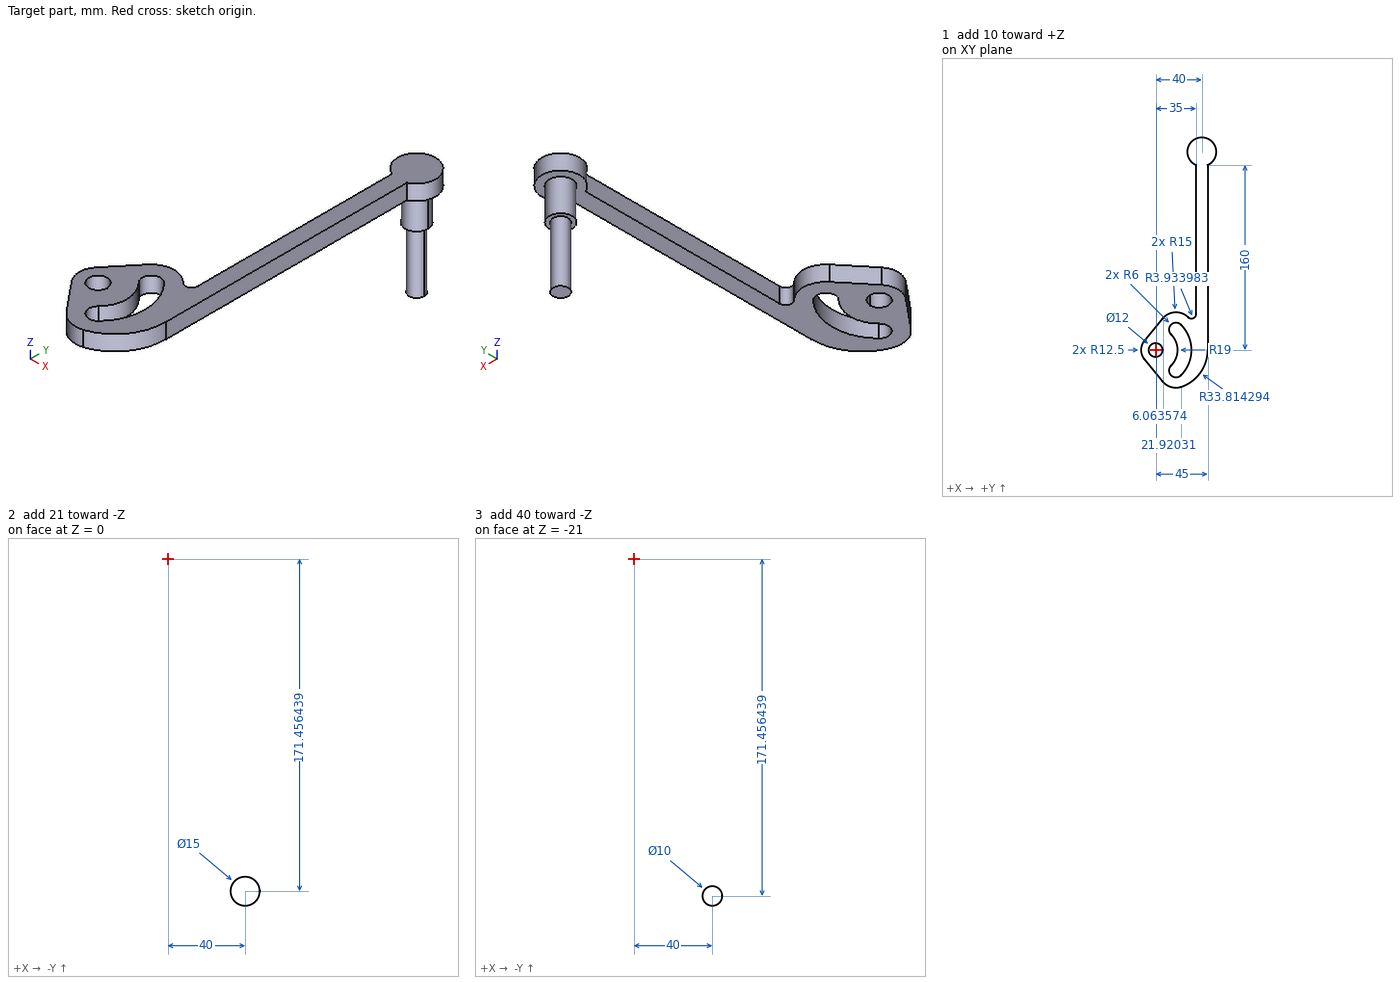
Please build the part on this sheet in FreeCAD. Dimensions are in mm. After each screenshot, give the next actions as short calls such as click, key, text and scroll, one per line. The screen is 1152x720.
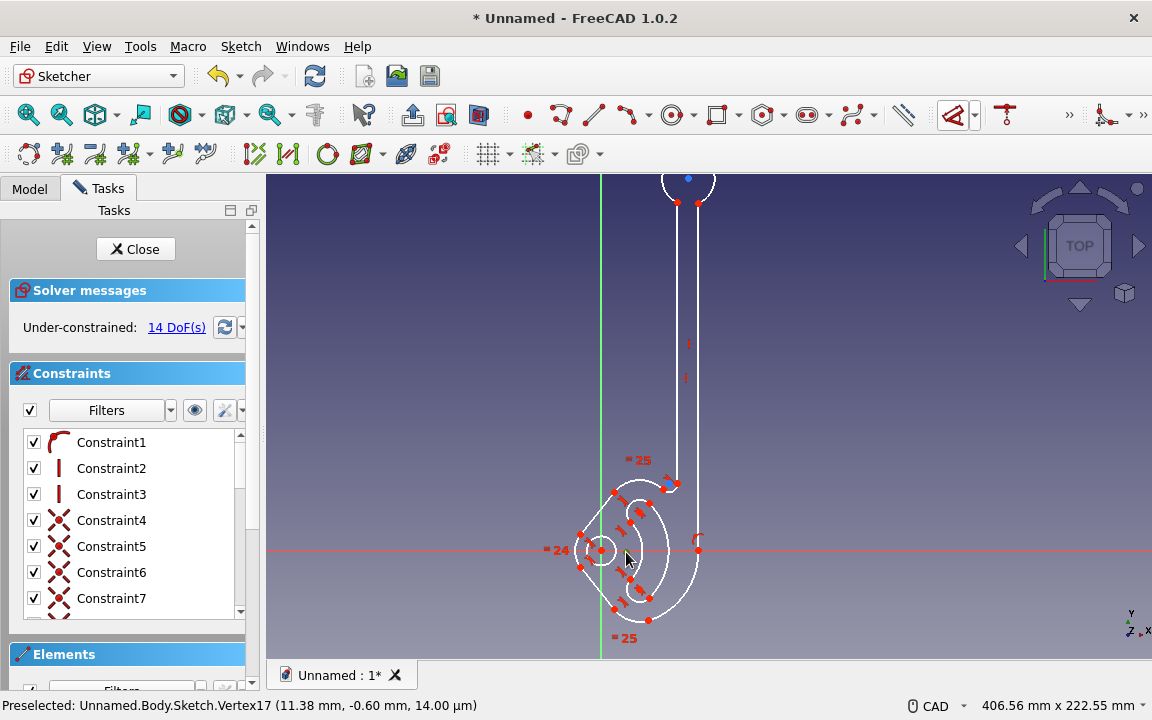
click(344, 551)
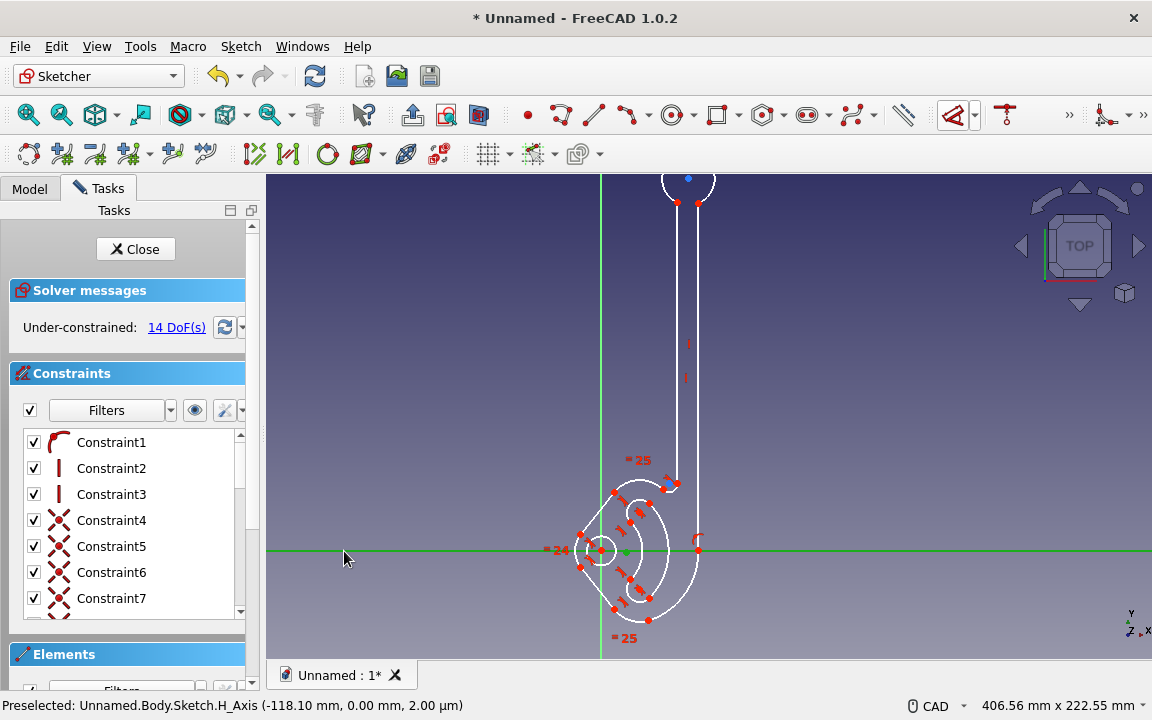
click(1005, 116)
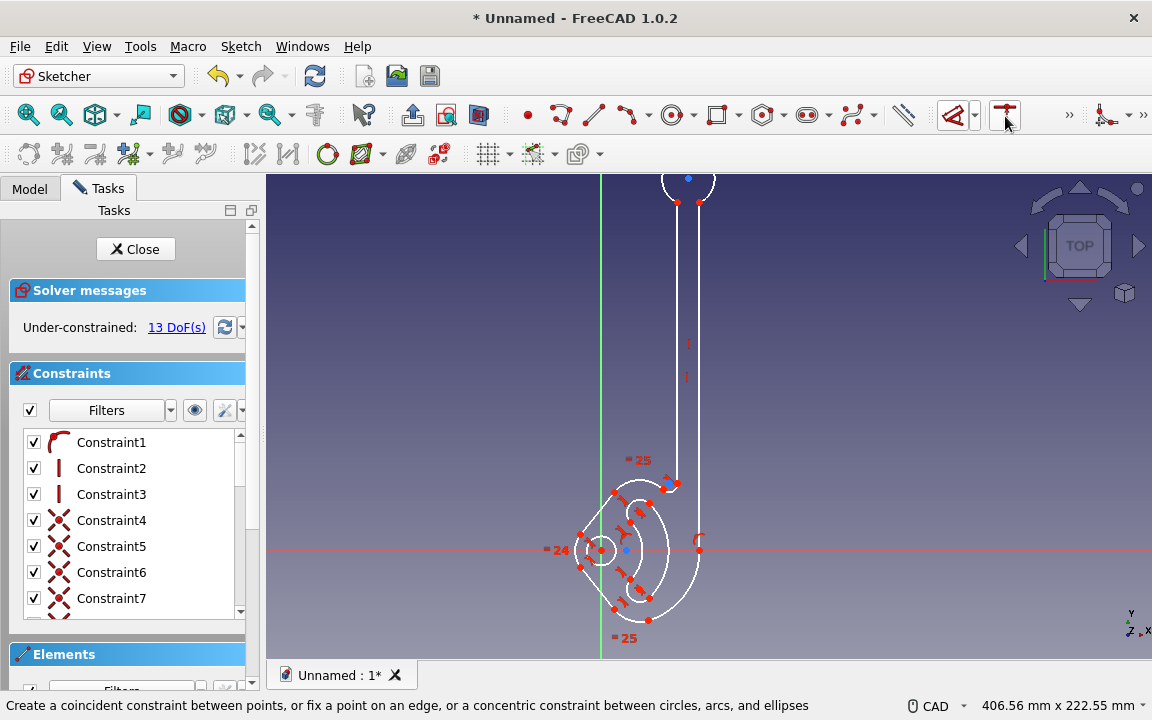
key(d)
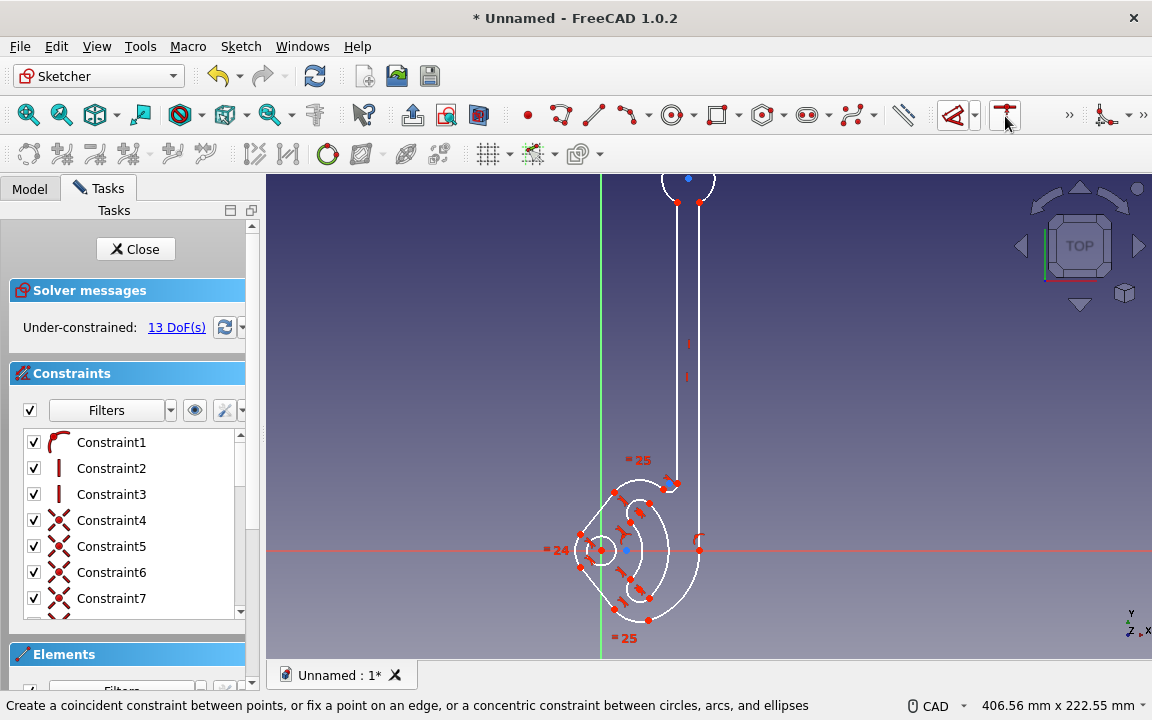
scroll(575, 551, up, 2)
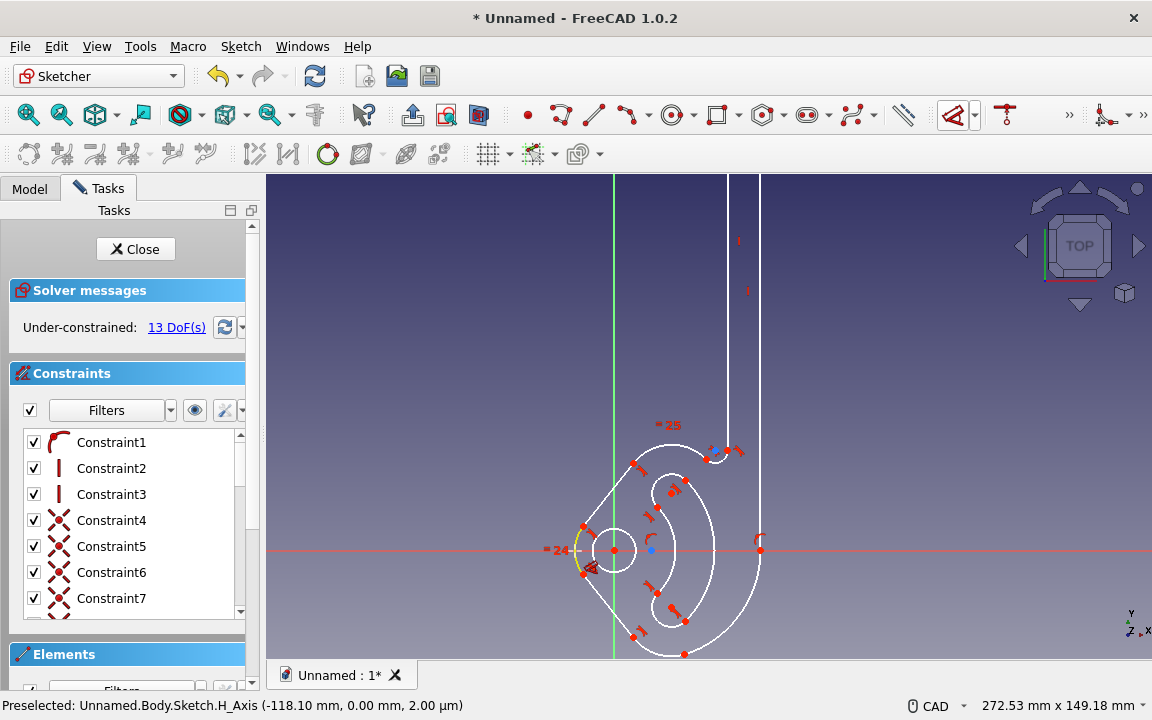
click(575, 551)
click(551, 517)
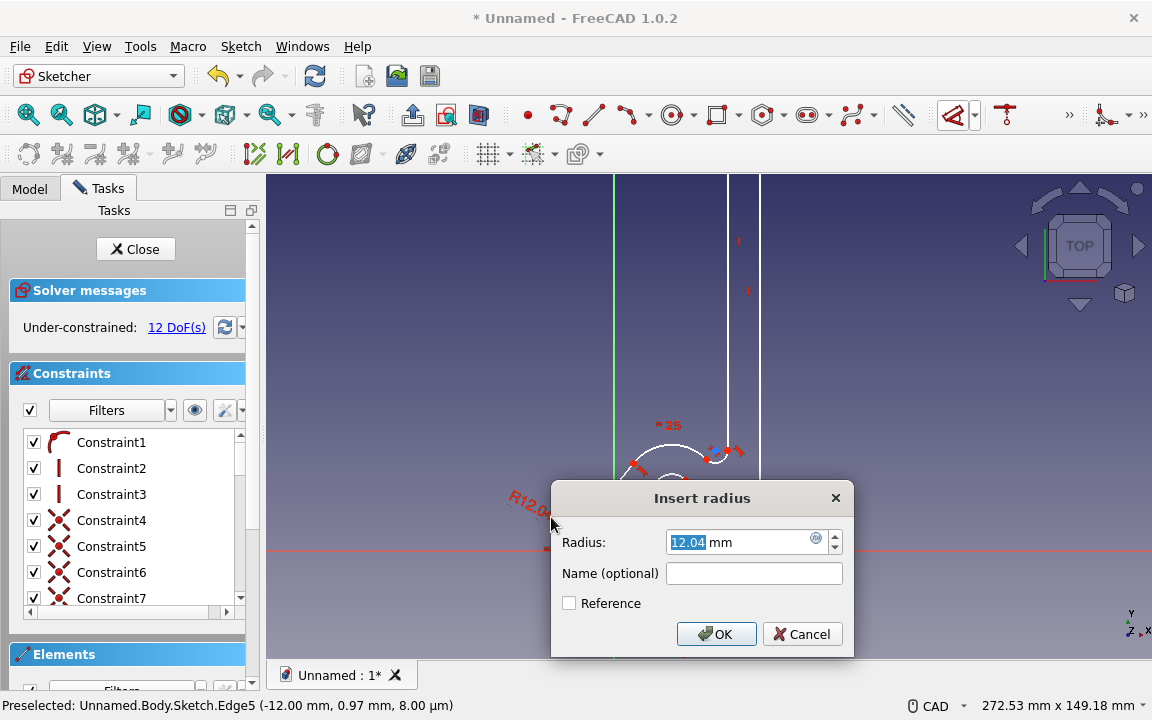
text(12.5)
key(Return)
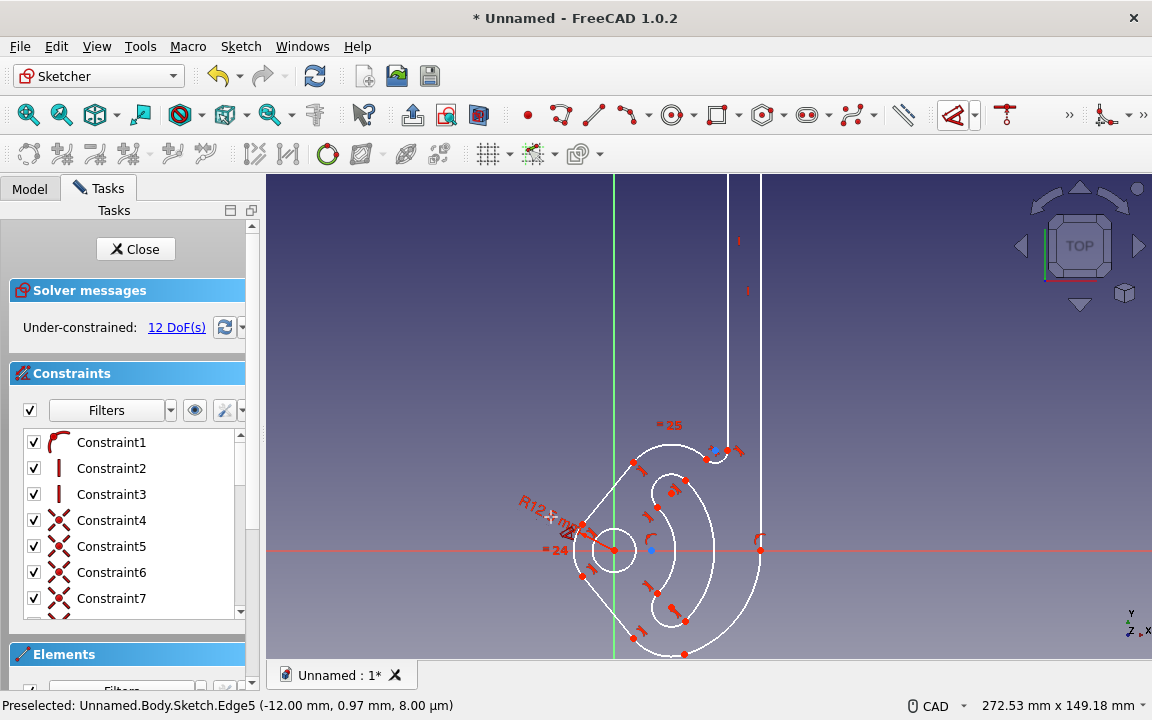
scroll(619, 509, down, 4)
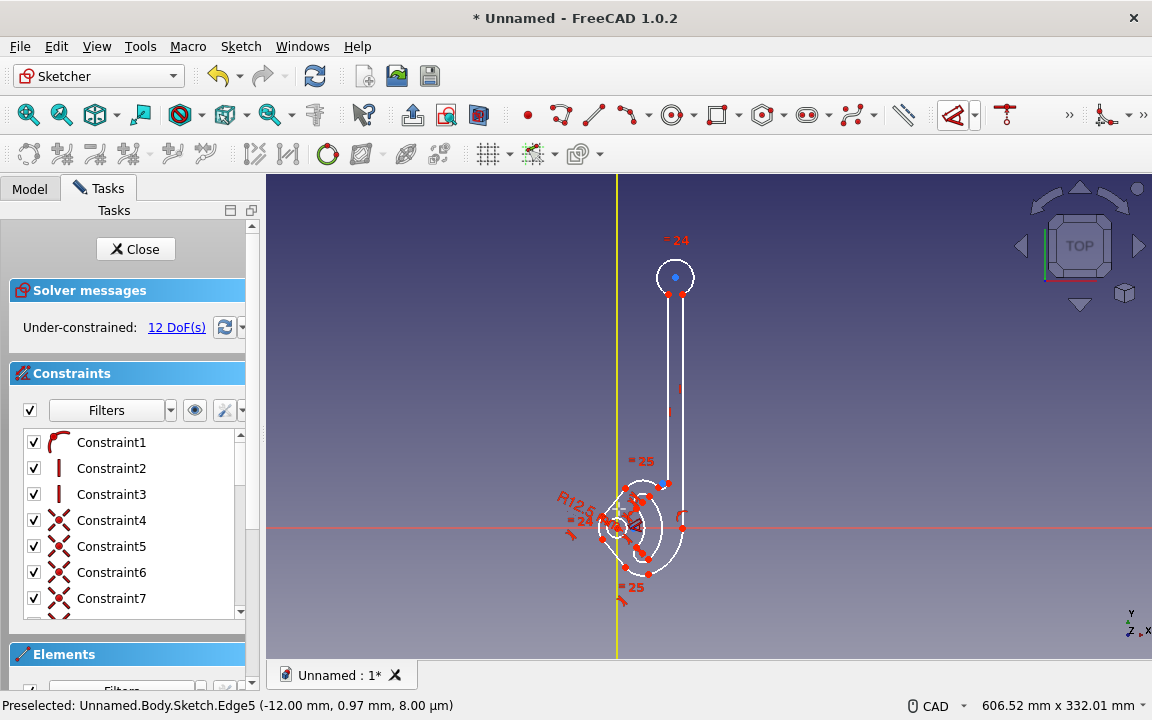
scroll(631, 573, up, 3)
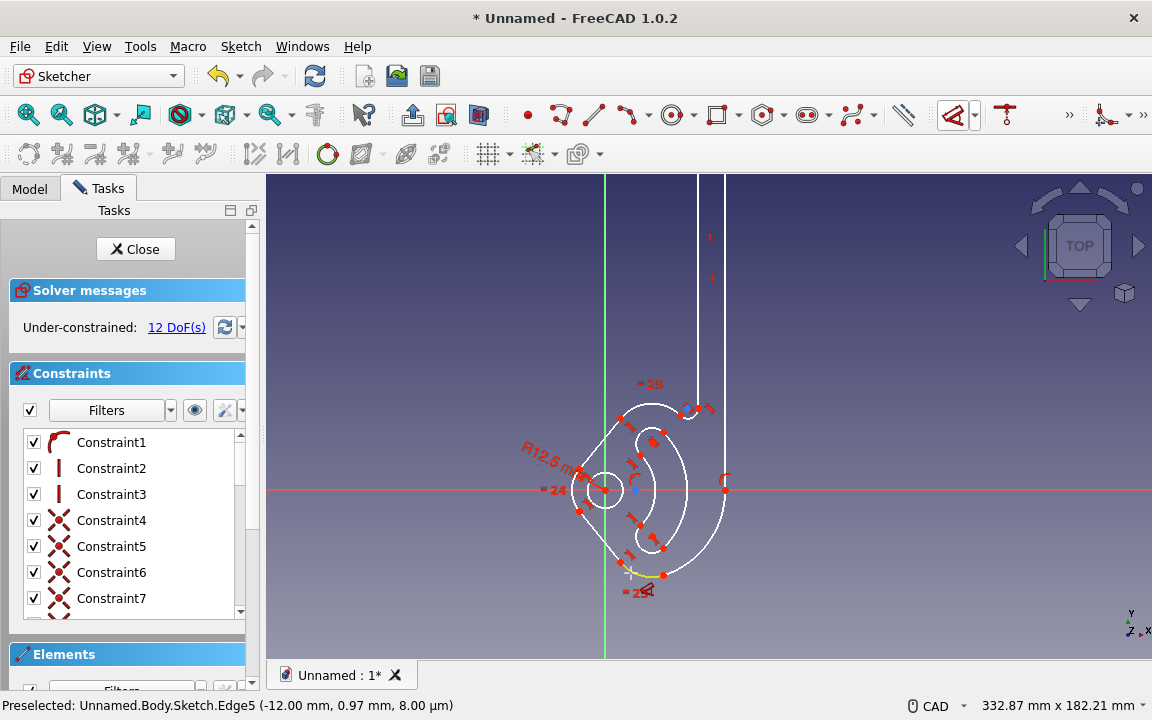
click(631, 572)
click(589, 574)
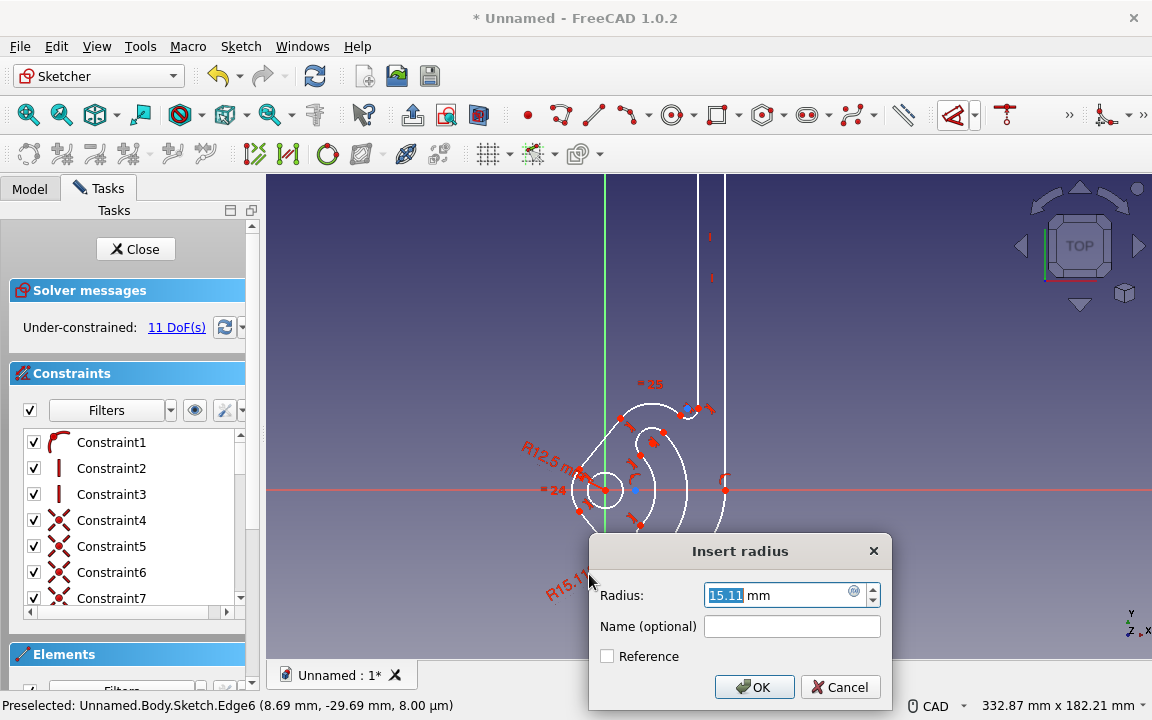
text(15)
key(Return)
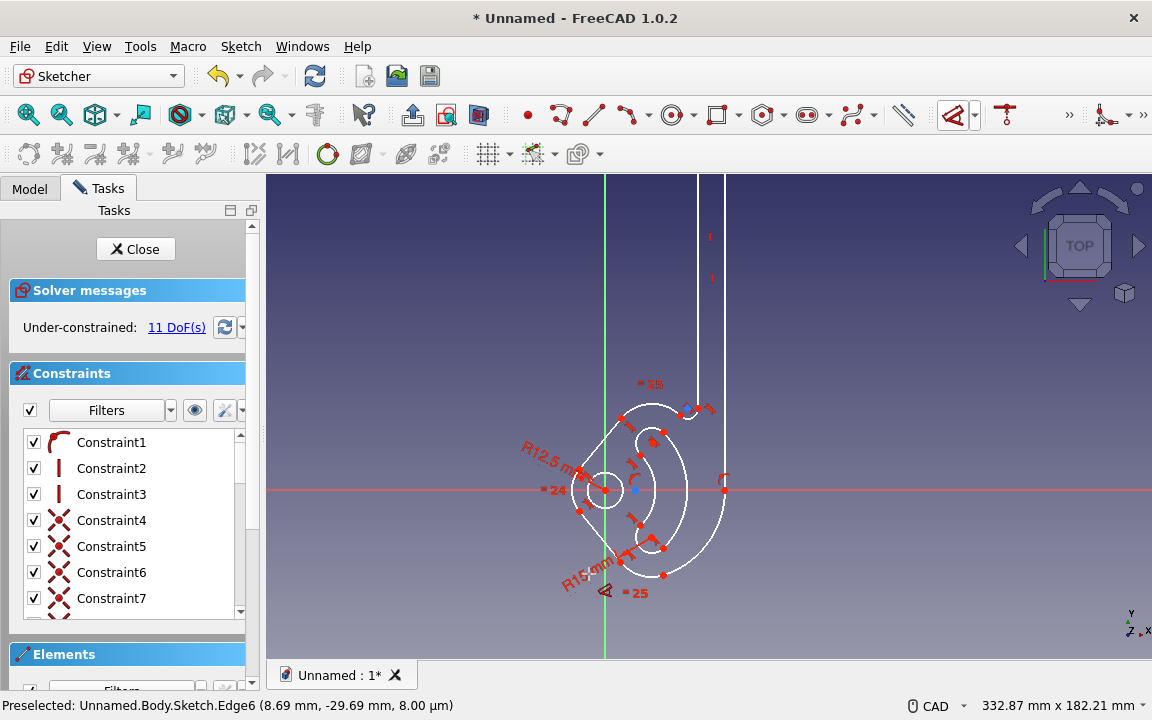
click(693, 559)
click(714, 584)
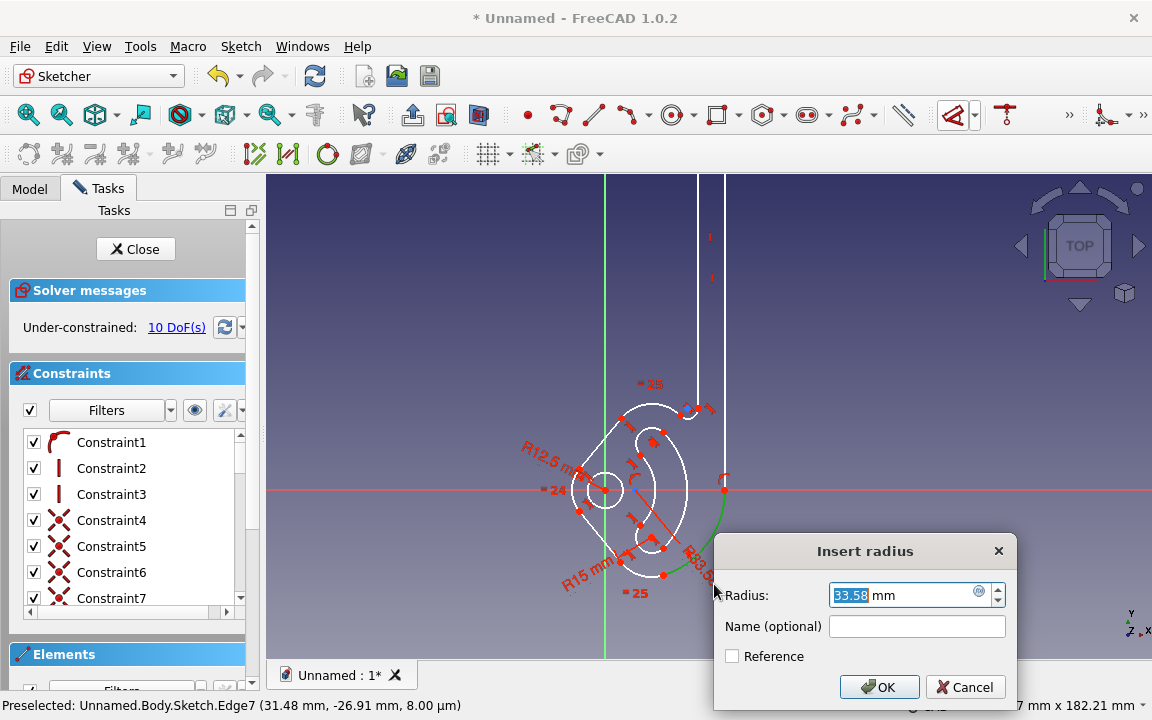
text(33.814294)
key(Return)